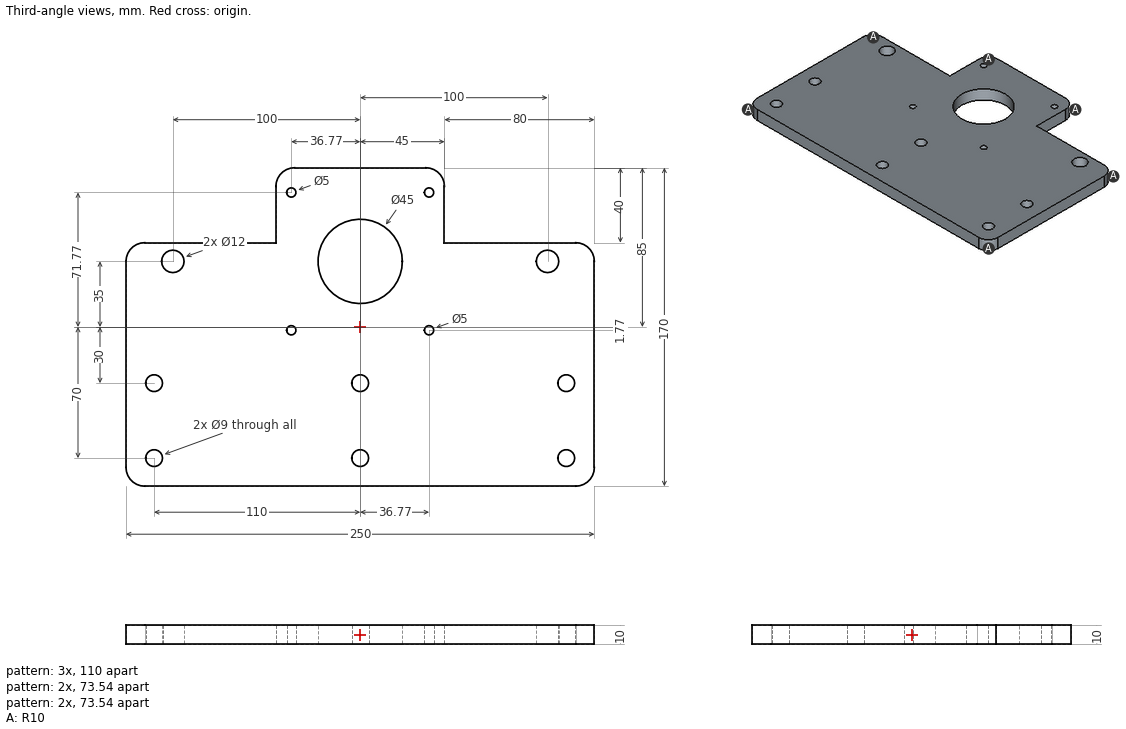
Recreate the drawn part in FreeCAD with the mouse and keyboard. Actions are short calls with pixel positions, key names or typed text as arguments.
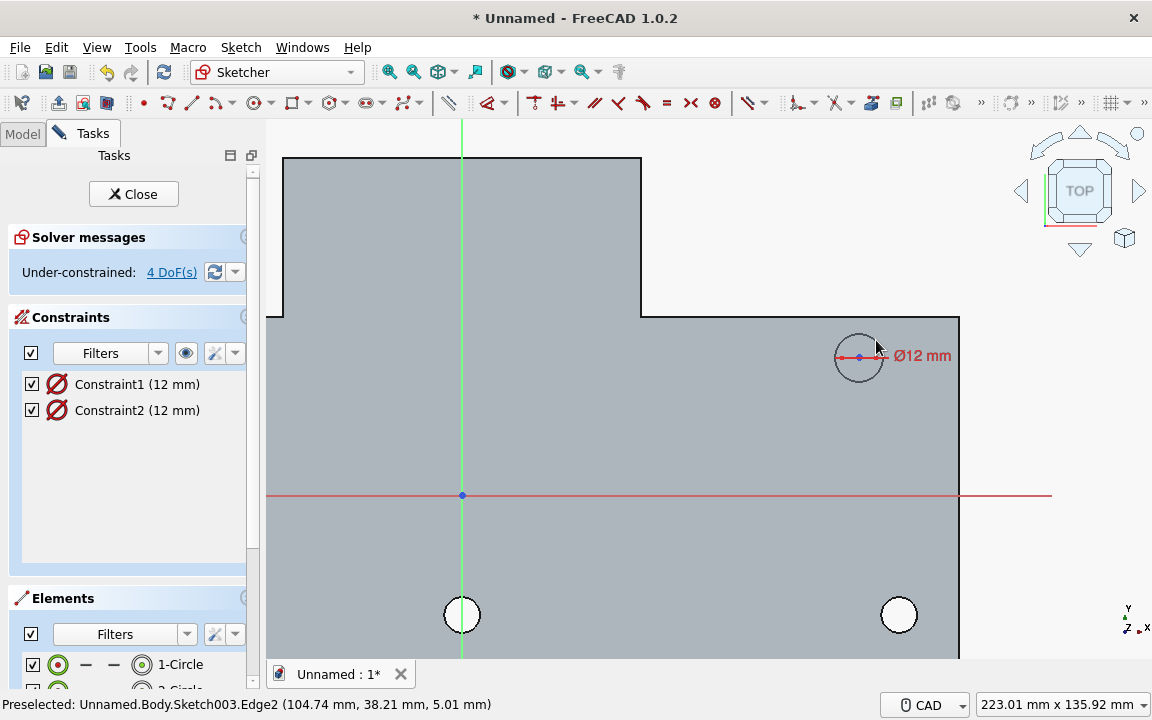
scroll(857, 358, down, 3)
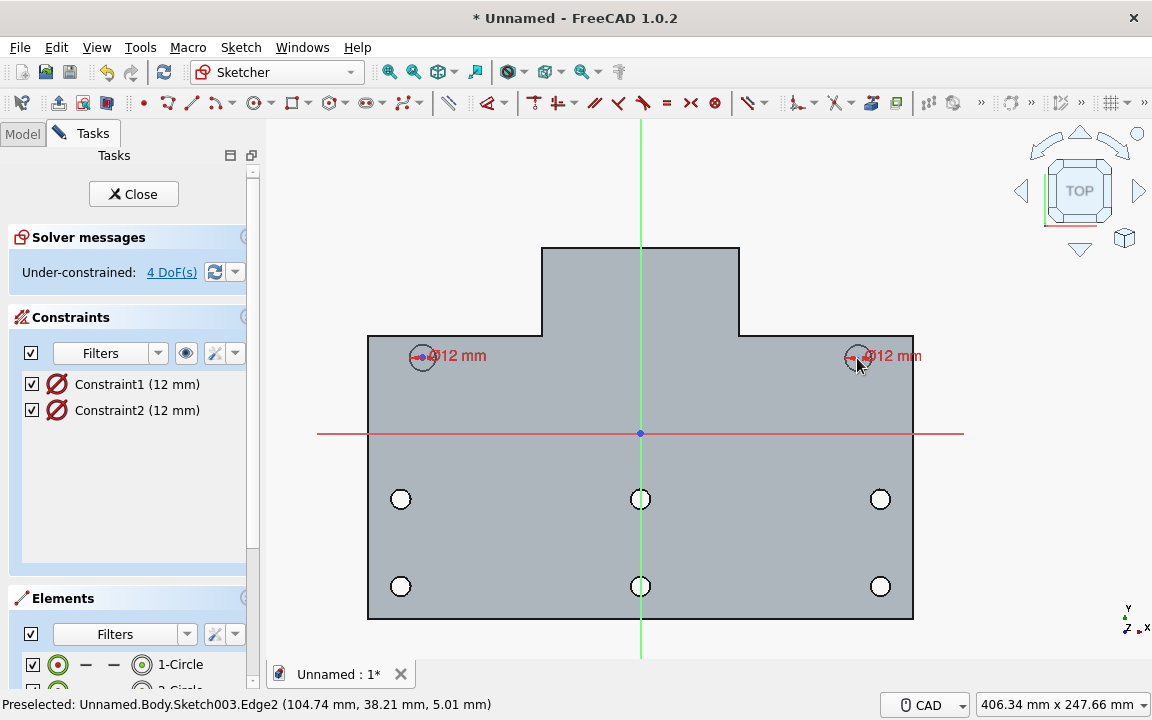
click(423, 358)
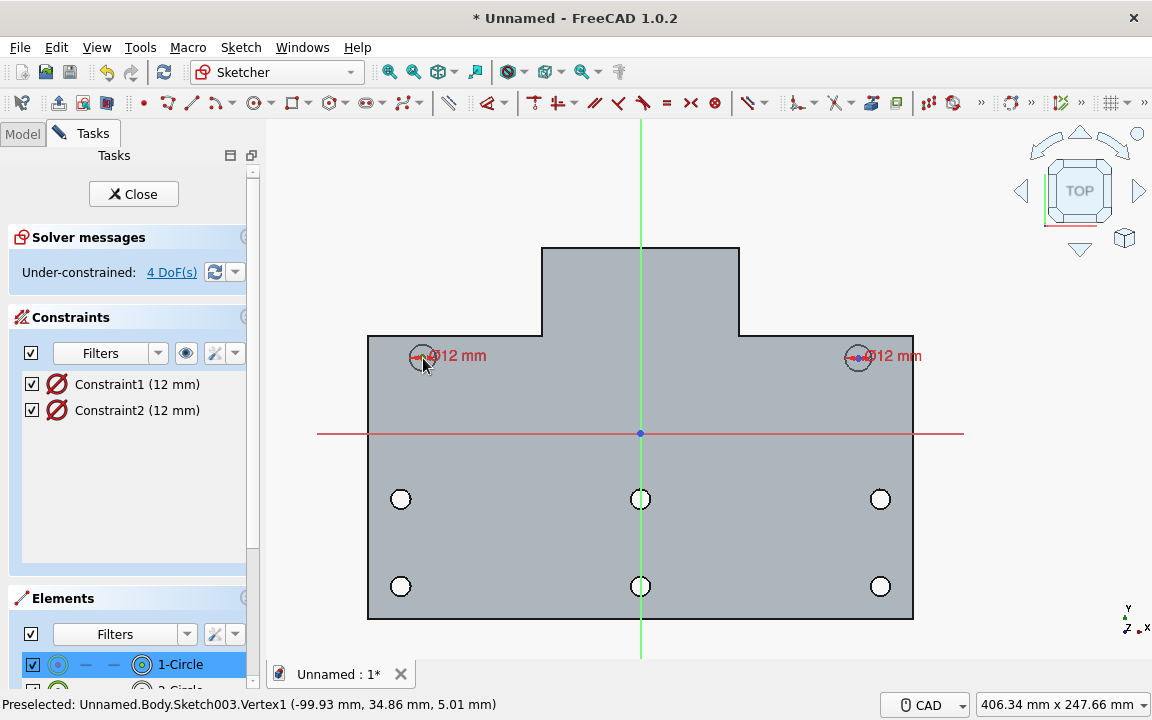
click(858, 358)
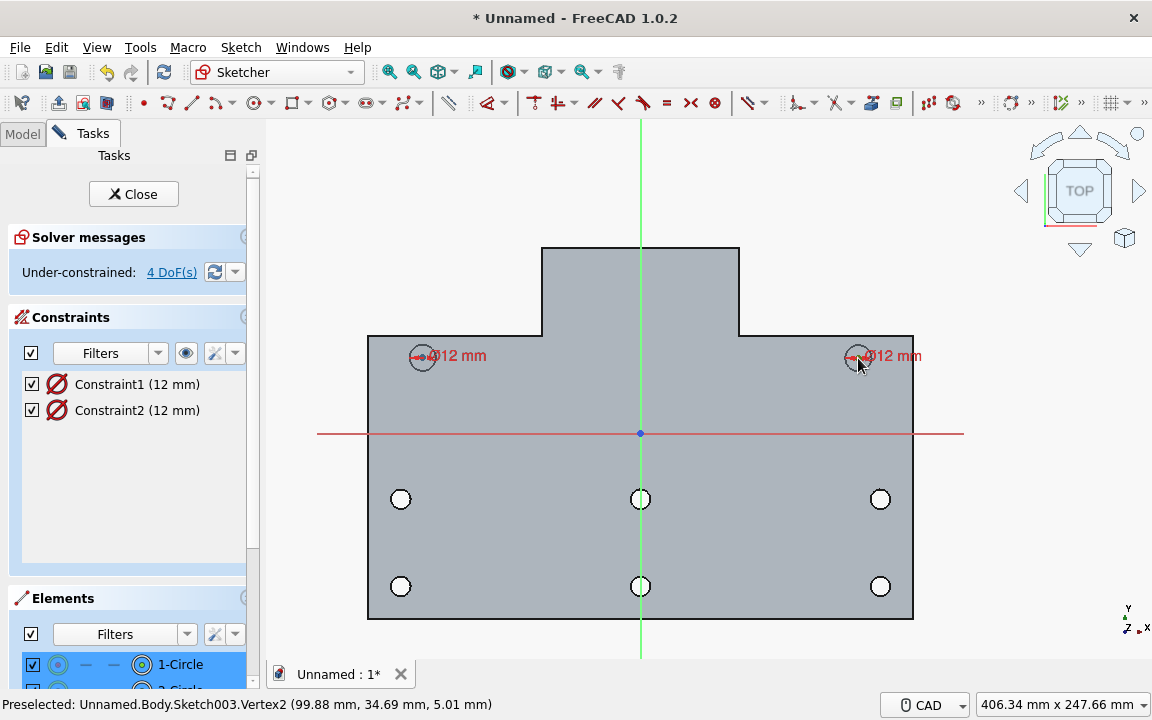
key(h)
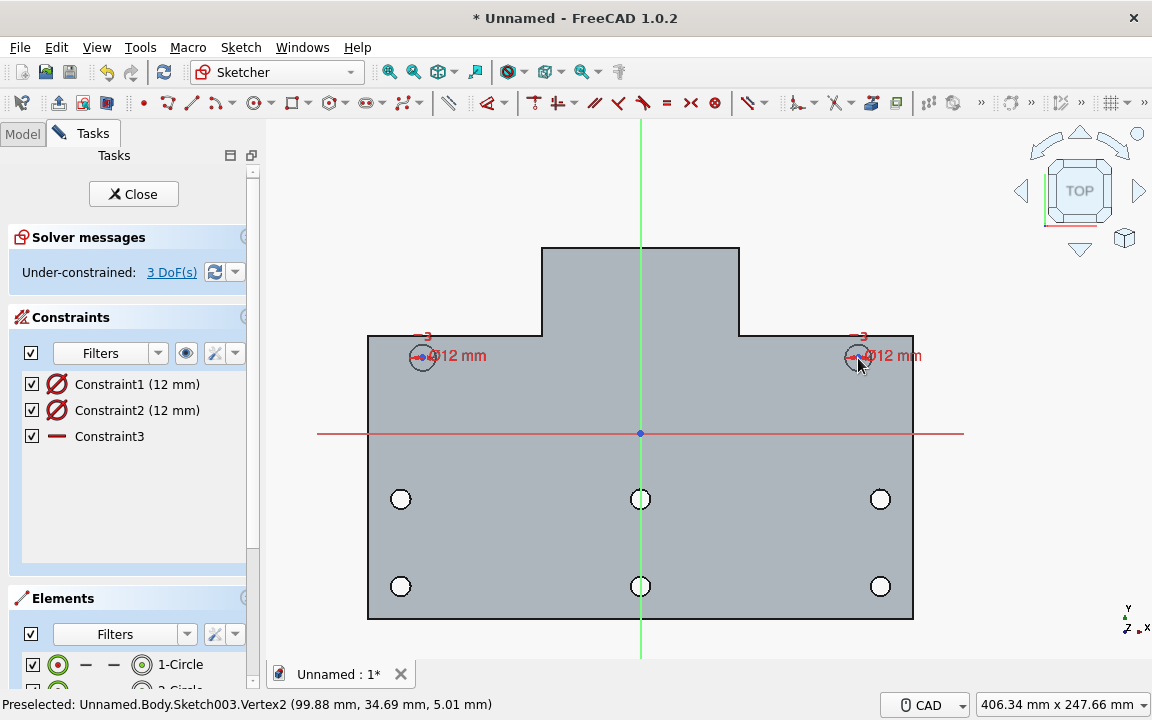
key(d)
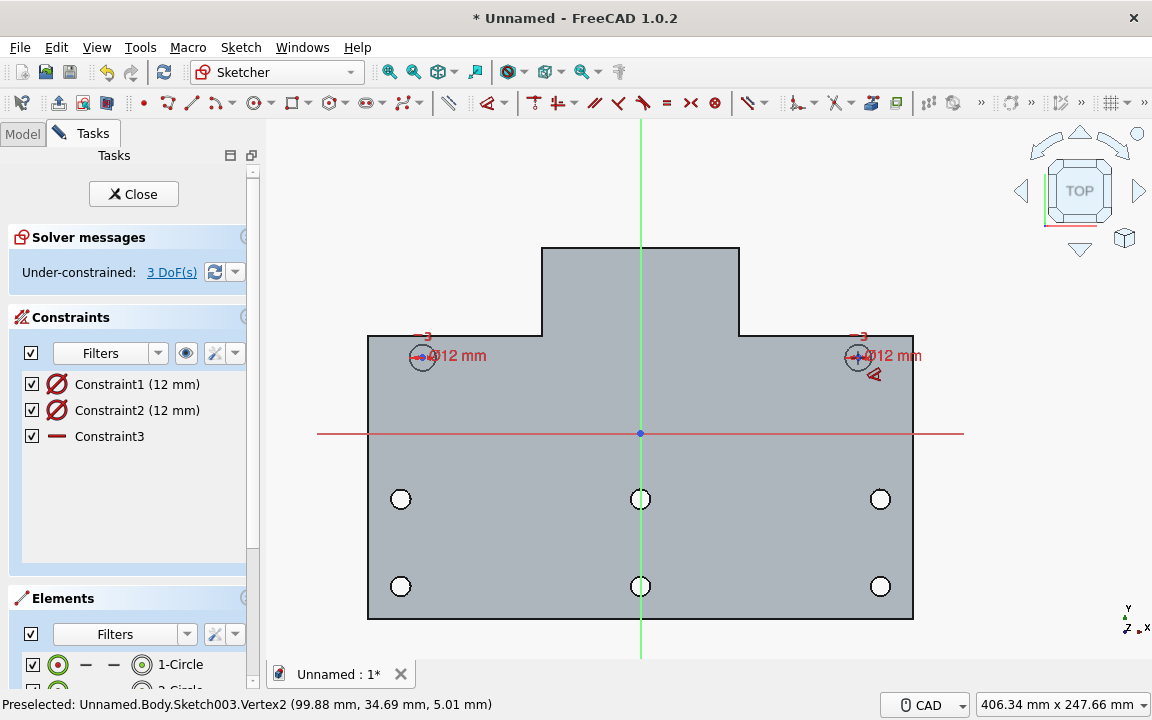
click(423, 358)
click(389, 396)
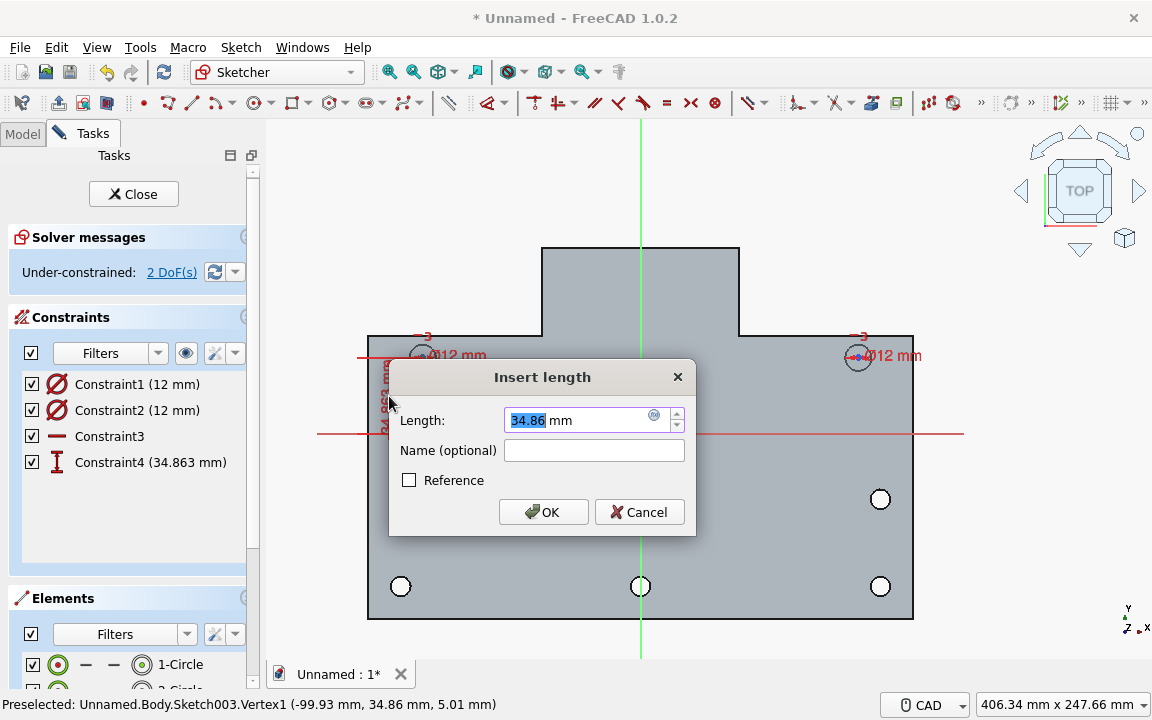
text(35)
key(Return)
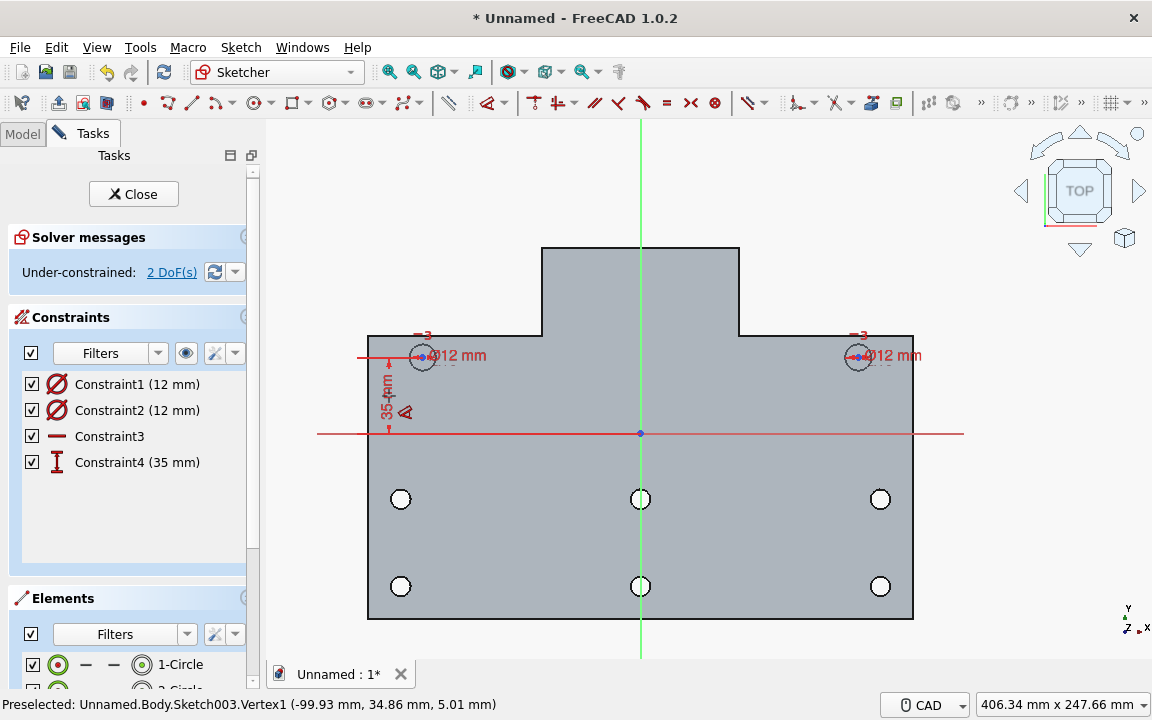
click(423, 358)
click(532, 468)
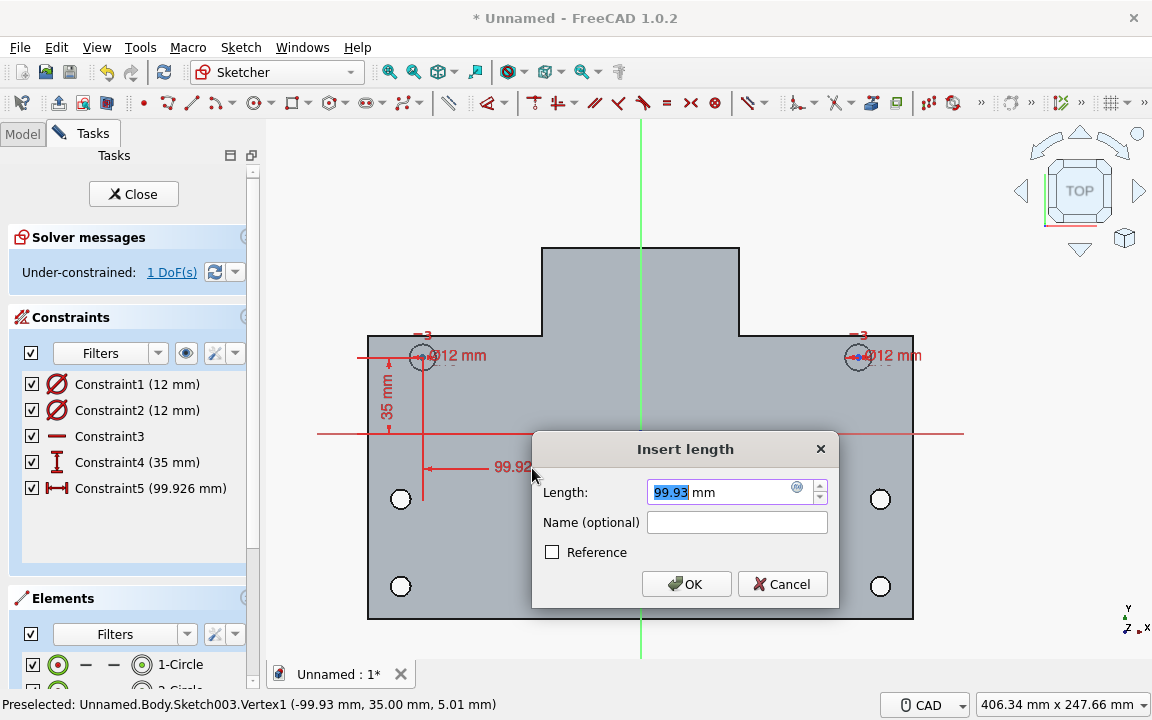
text(100)
key(Return)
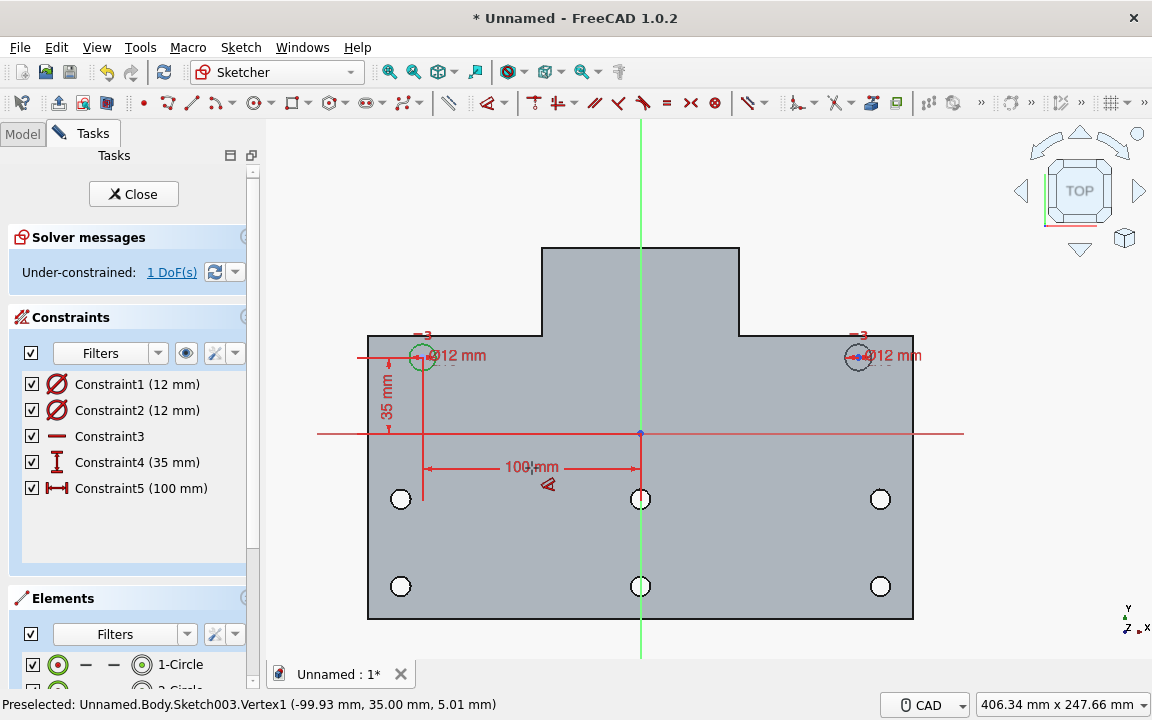
click(858, 358)
click(750, 468)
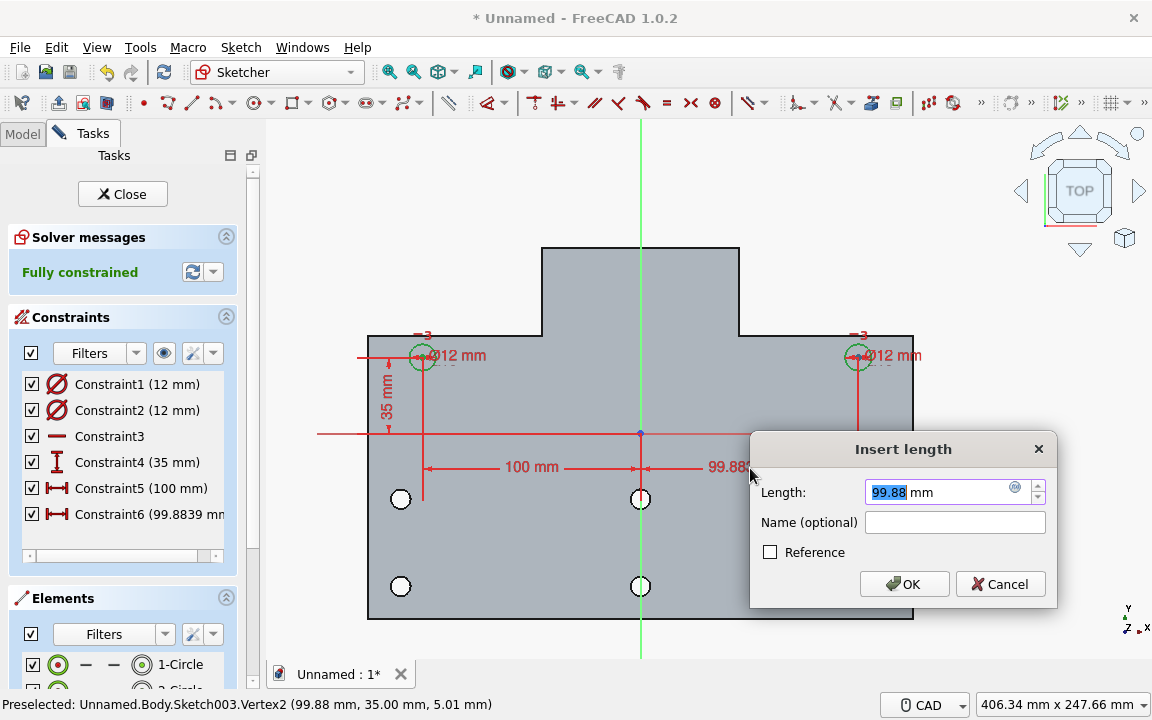
text(100)
key(Return)
key(Escape)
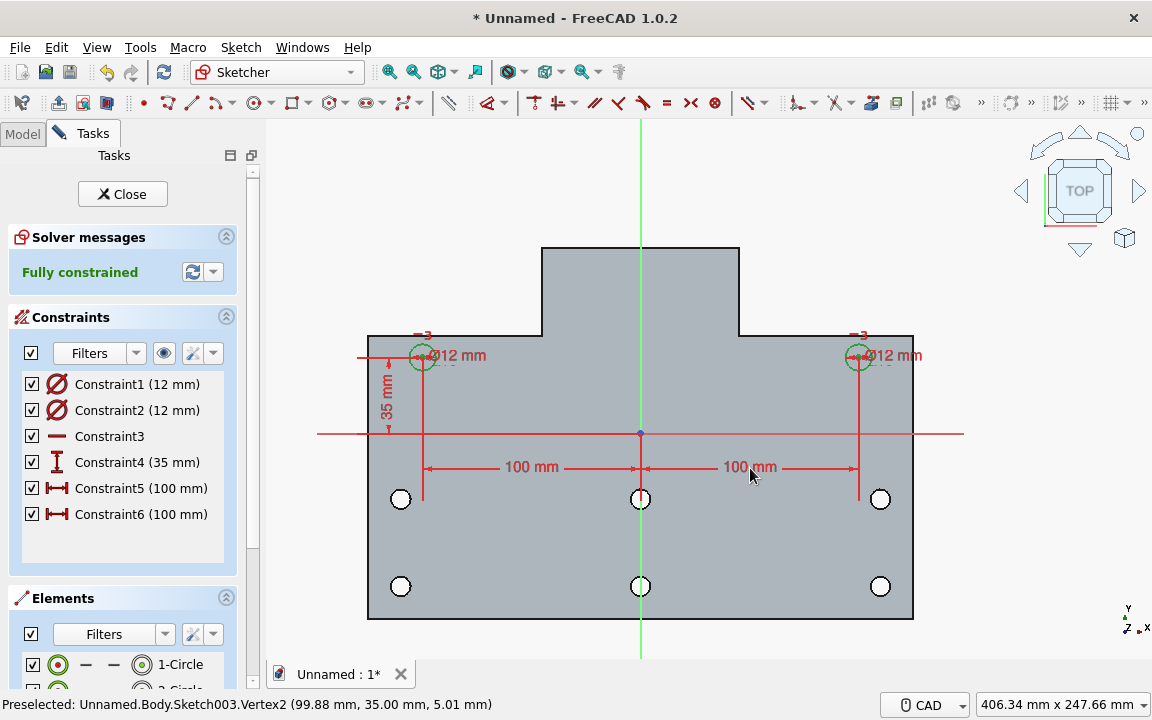
click(123, 194)